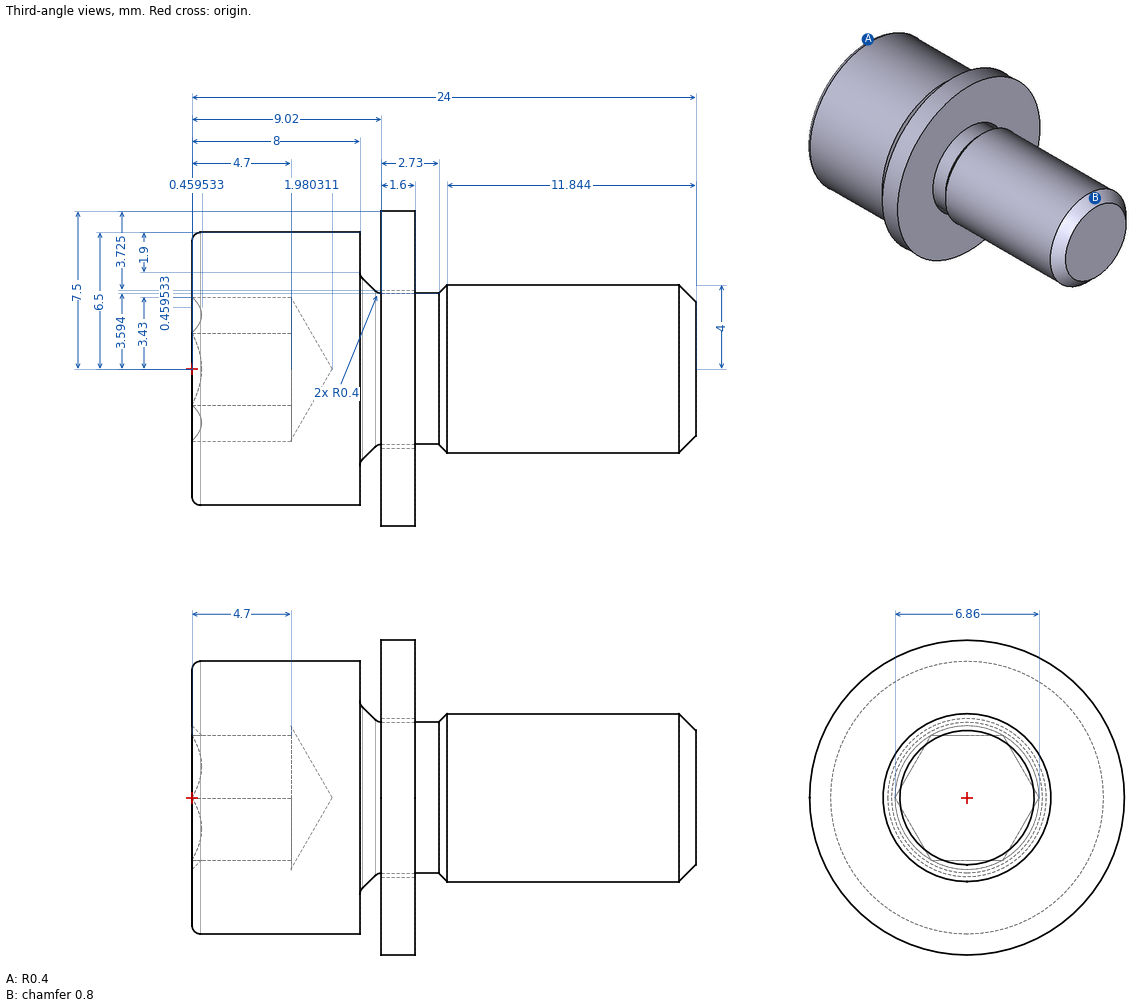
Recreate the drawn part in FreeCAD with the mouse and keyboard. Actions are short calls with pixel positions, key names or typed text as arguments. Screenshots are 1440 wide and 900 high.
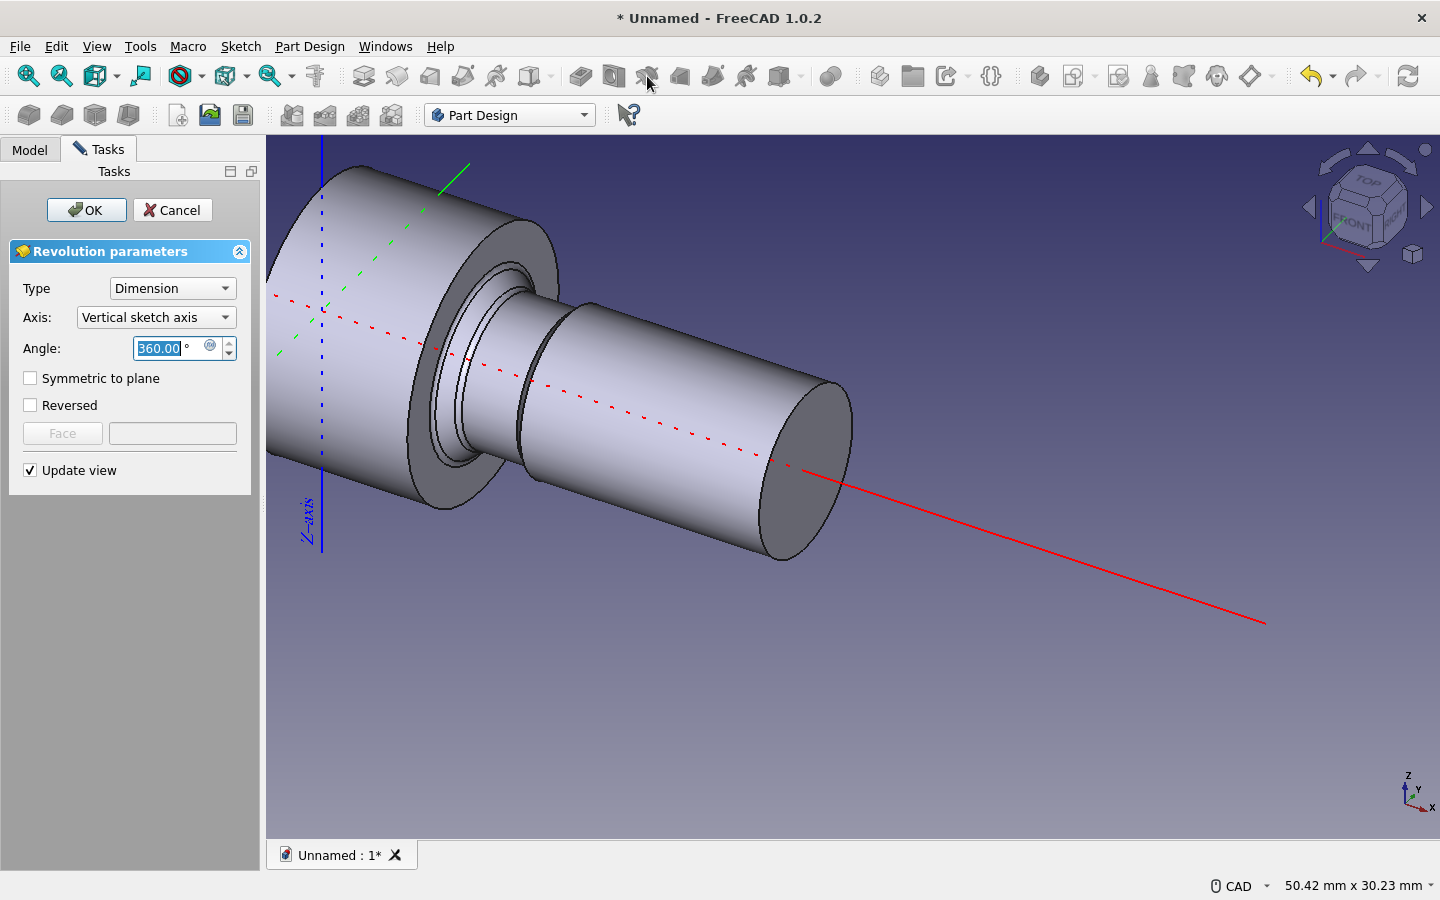
click(157, 318)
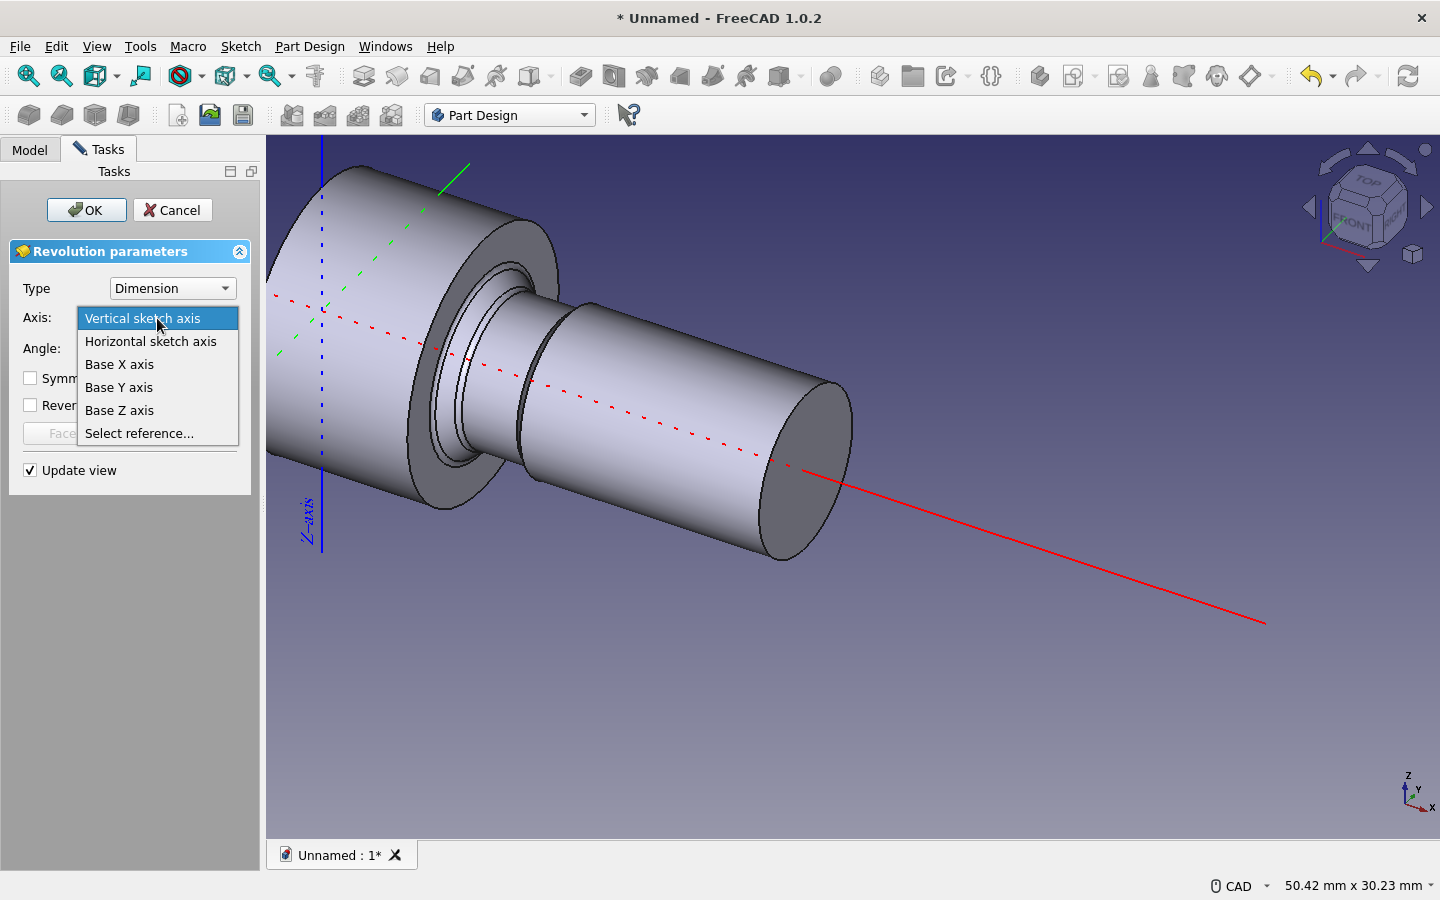
click(156, 342)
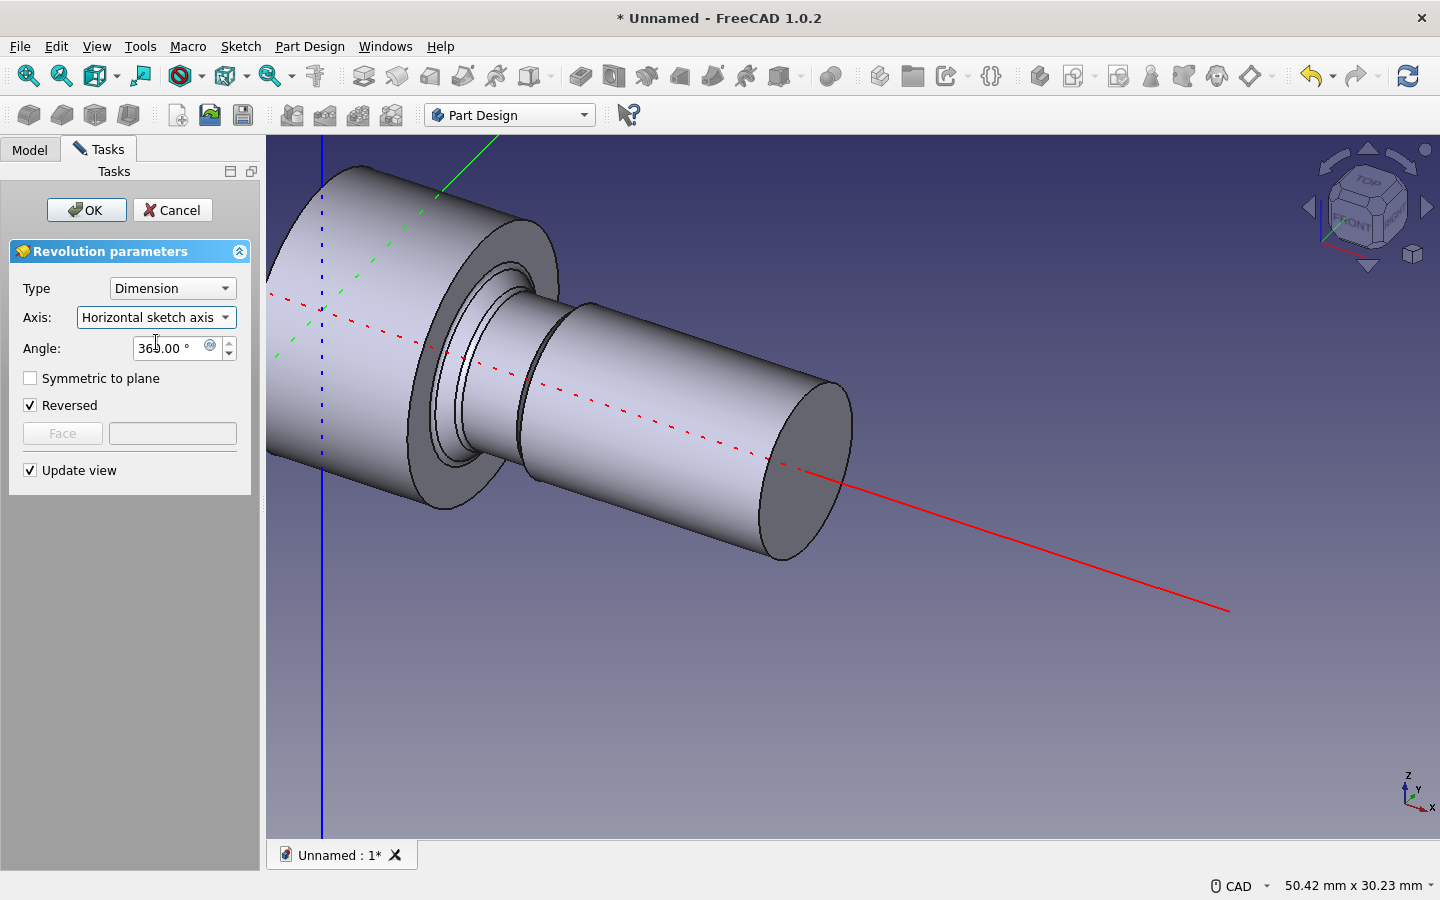
click(87, 210)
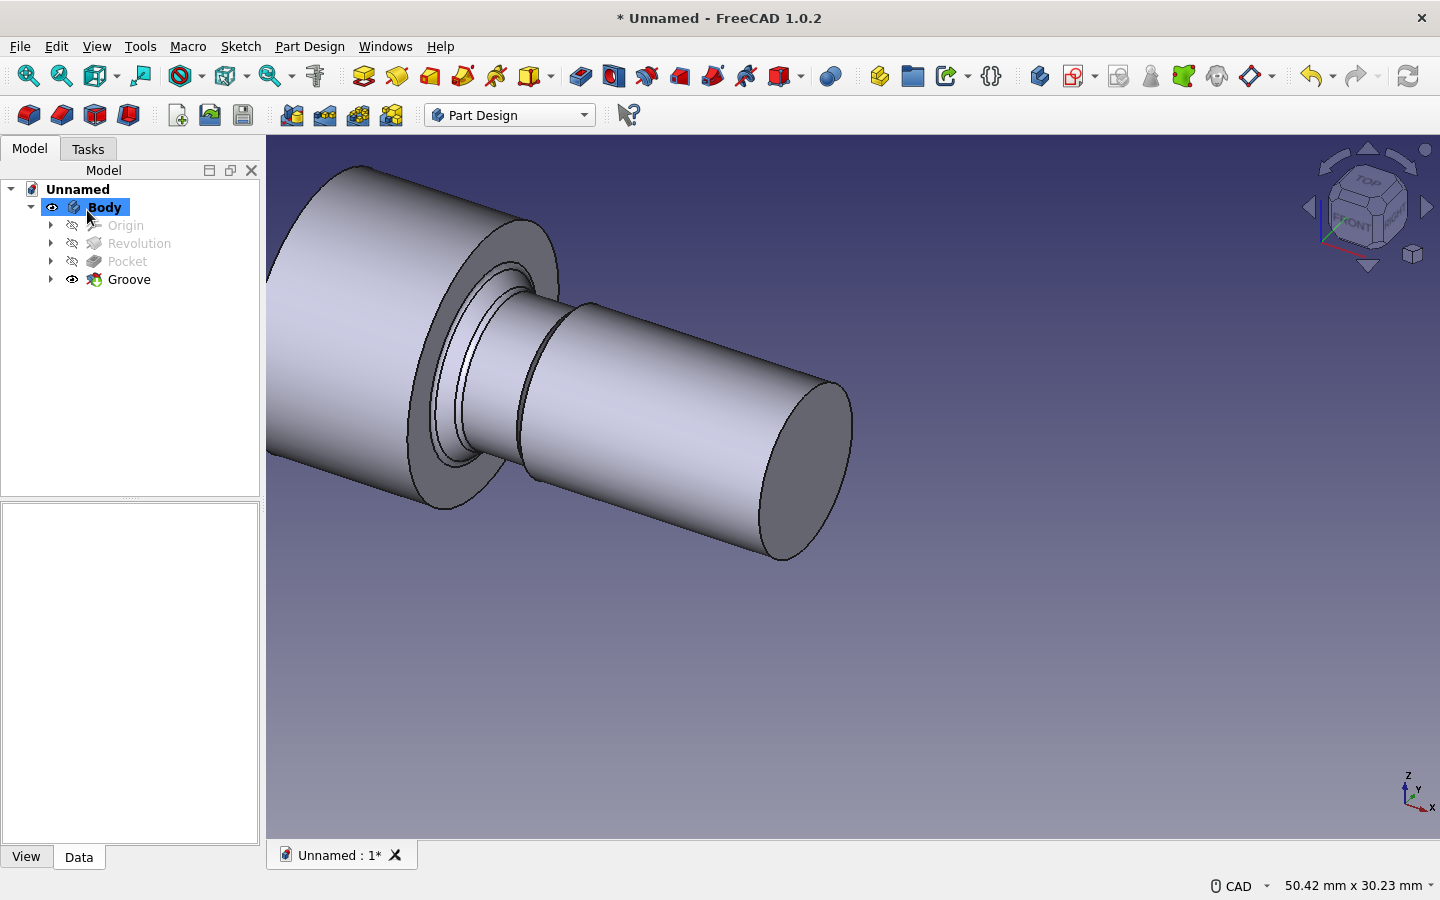
click(29, 76)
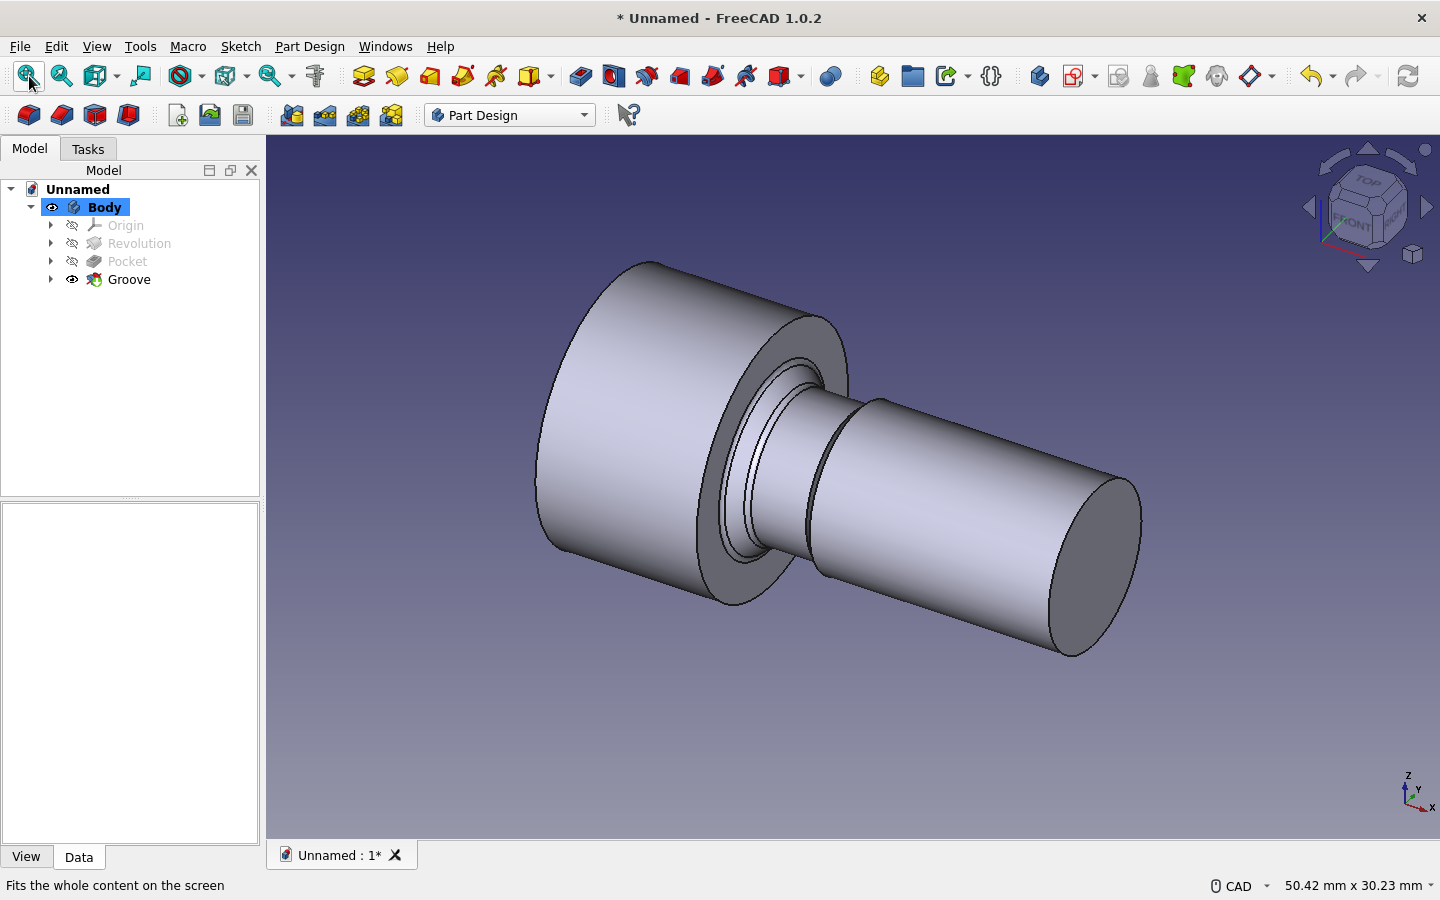
click(1072, 76)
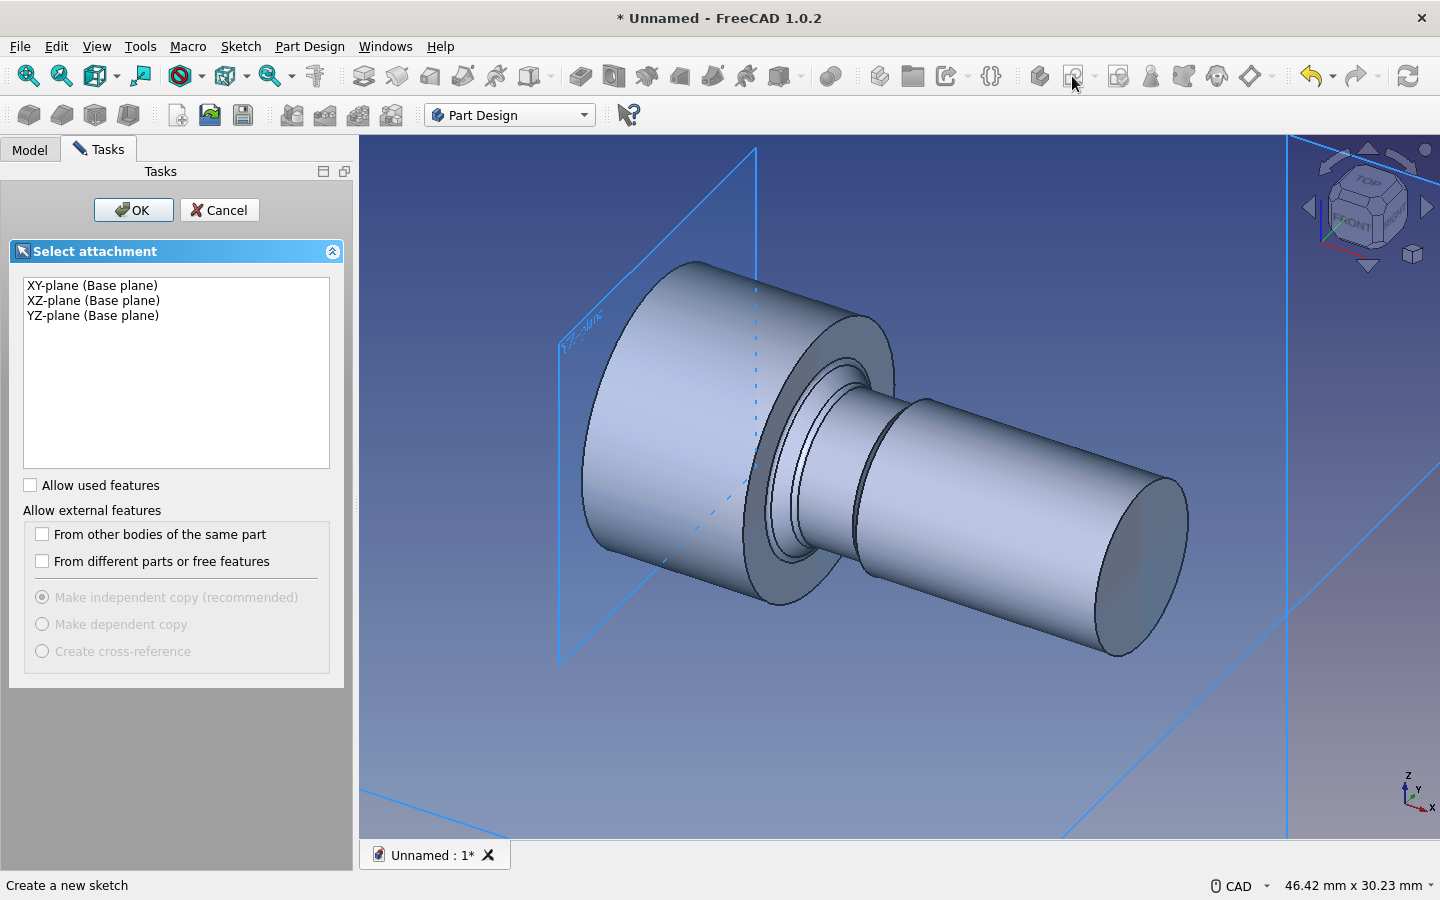
click(84, 286)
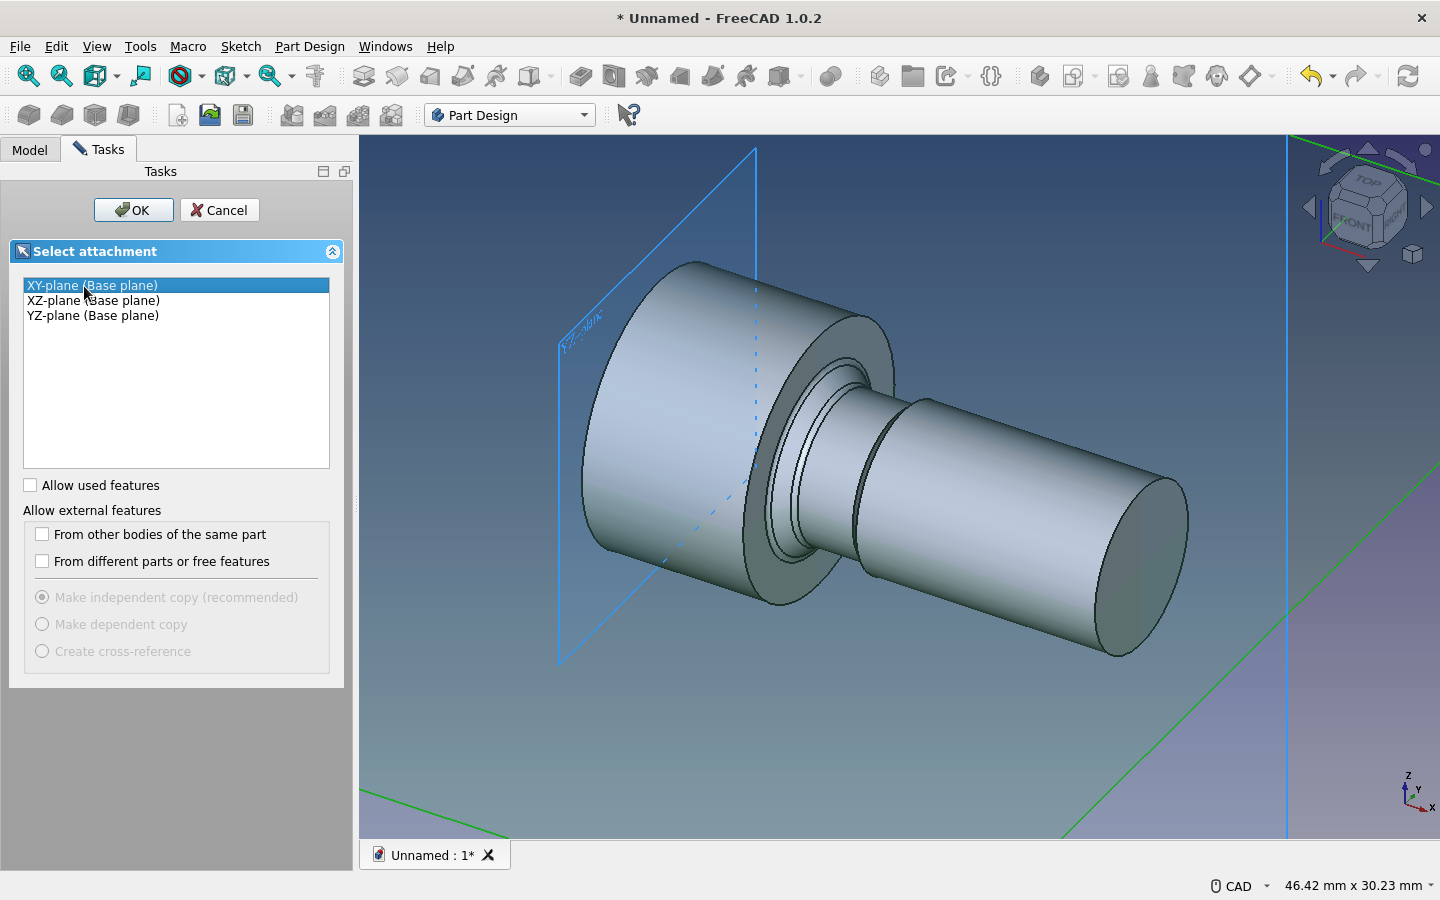
click(134, 210)